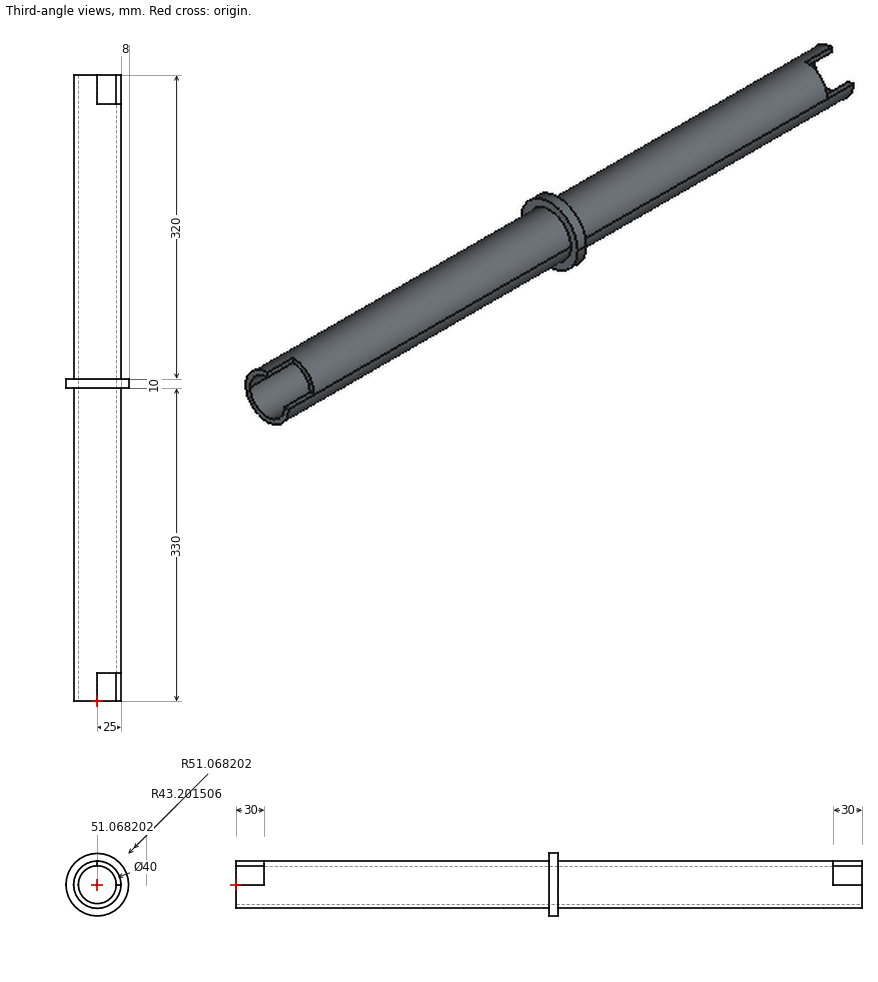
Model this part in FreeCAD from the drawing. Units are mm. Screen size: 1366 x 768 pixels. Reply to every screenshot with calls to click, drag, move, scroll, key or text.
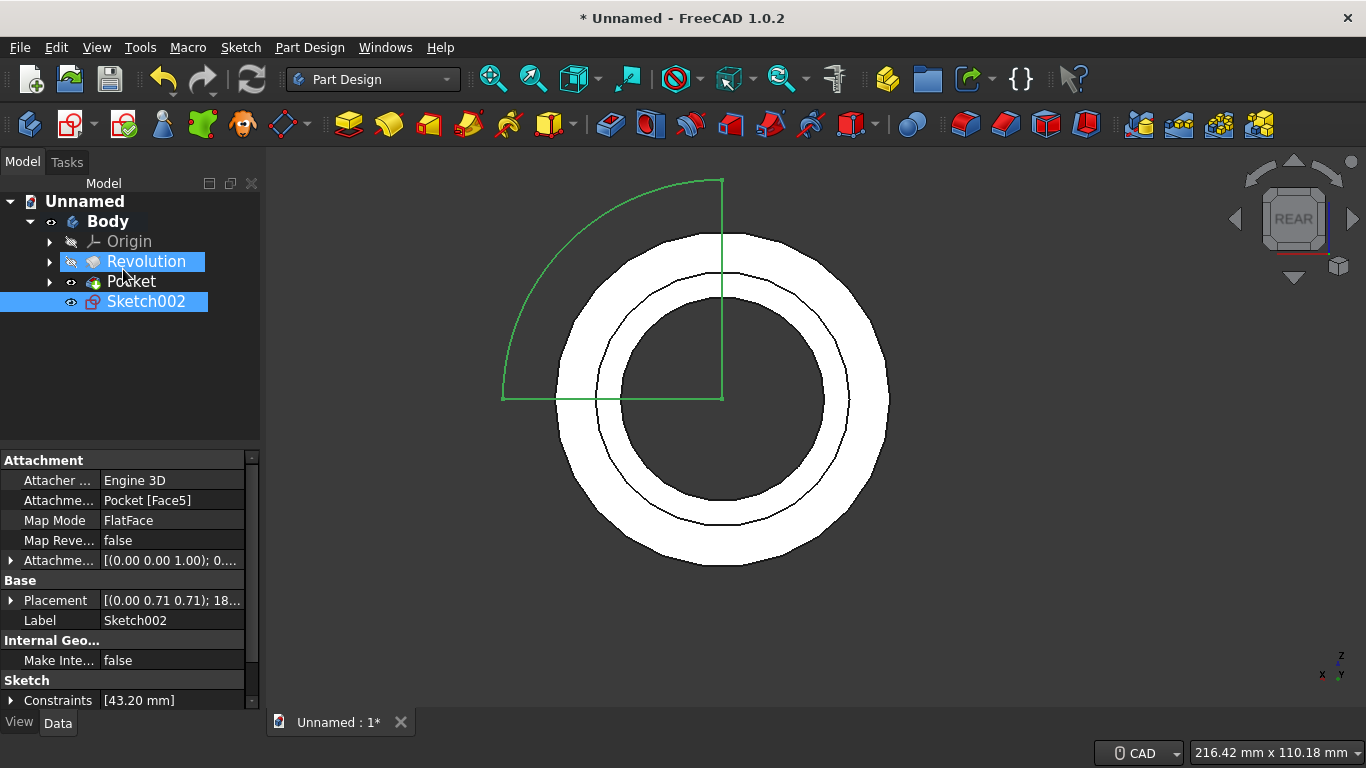
click(612, 124)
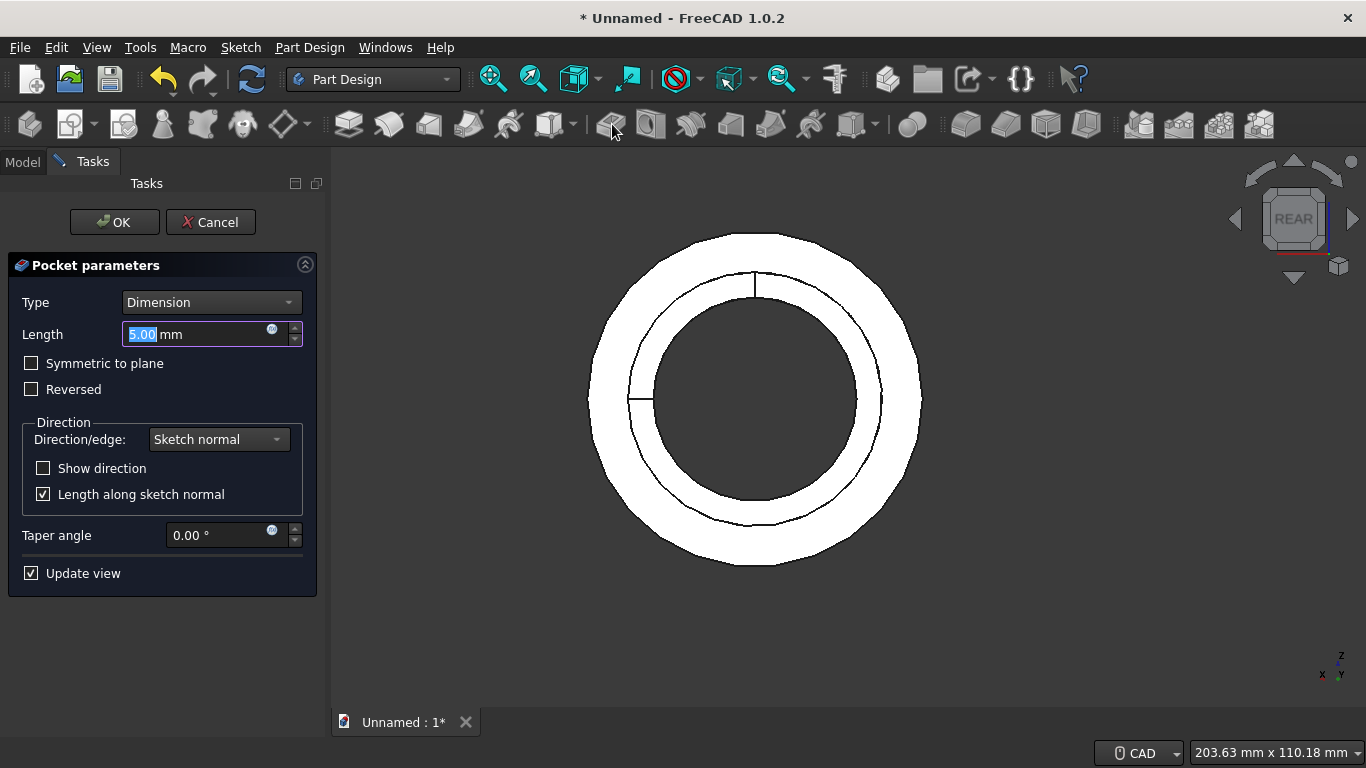
text(30)
key(Tab)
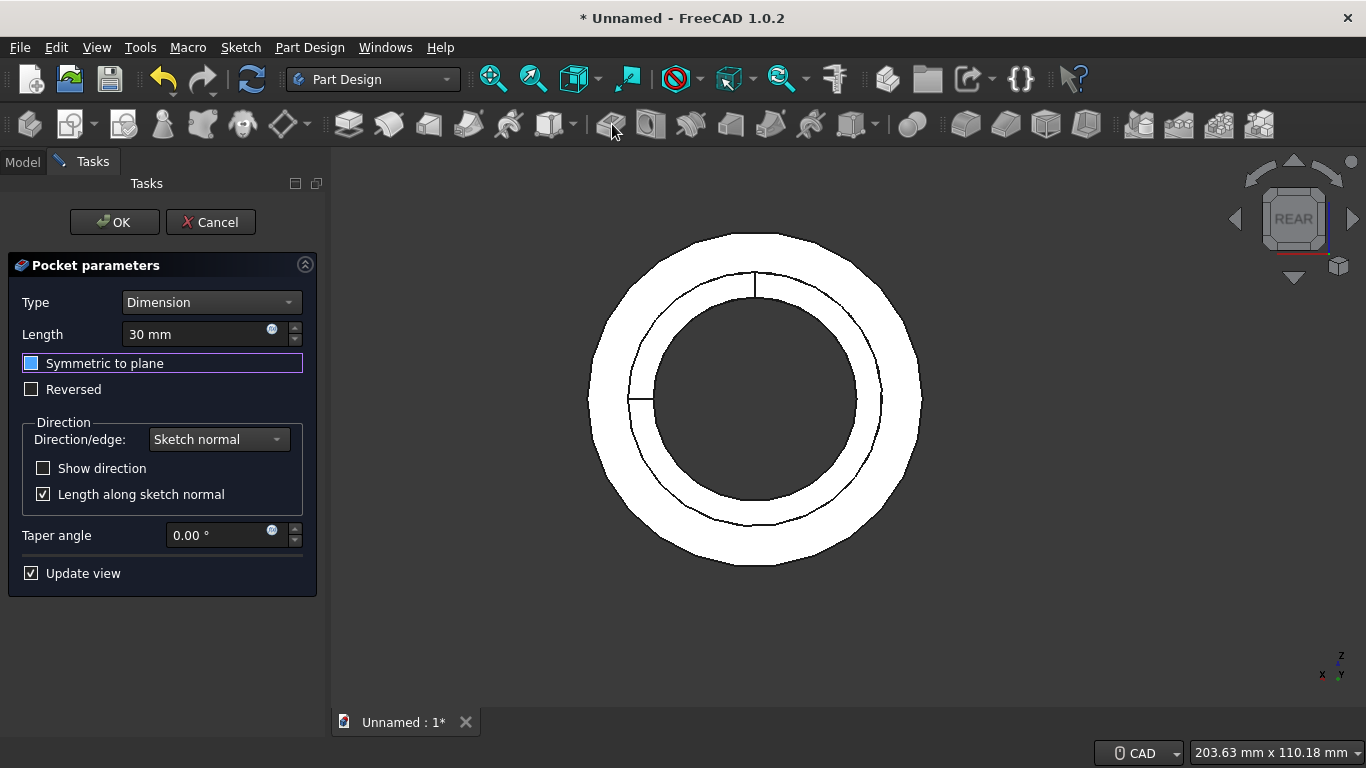
click(115, 222)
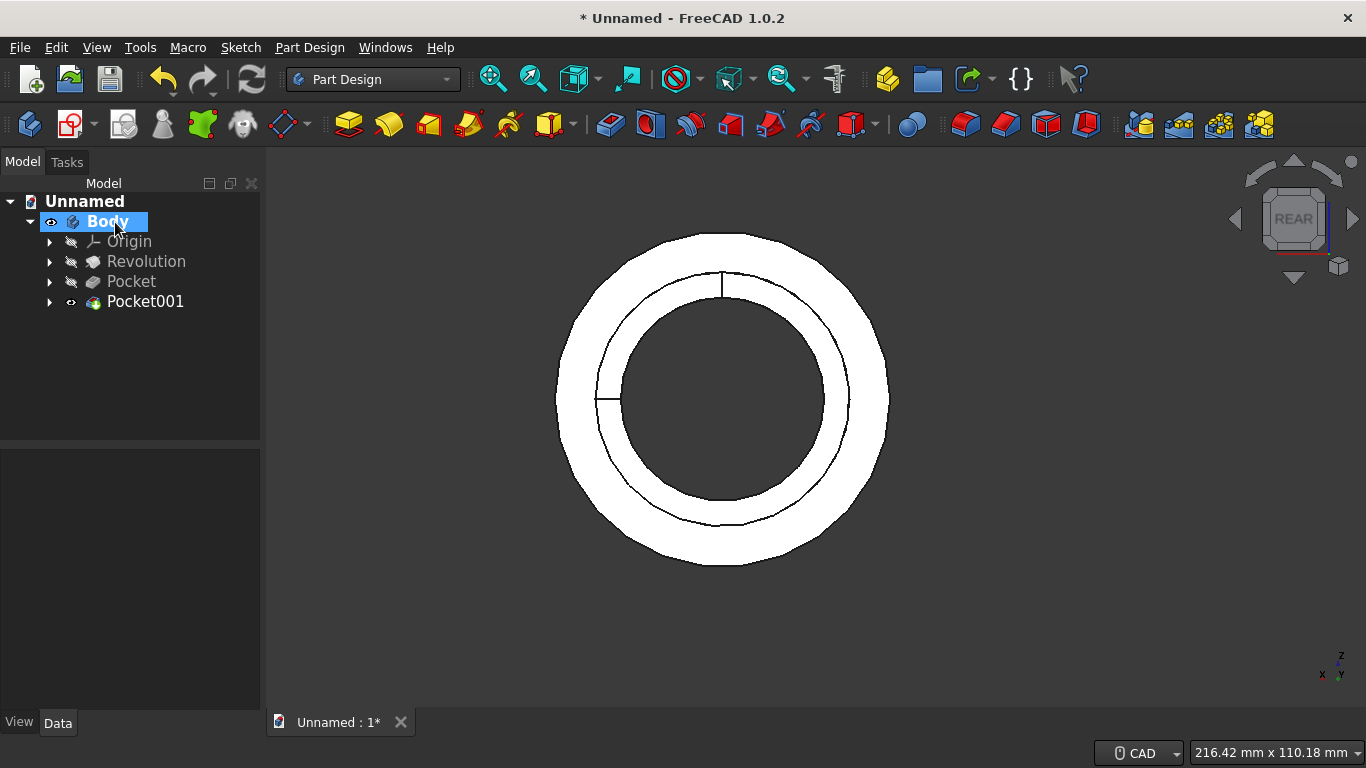
key(0)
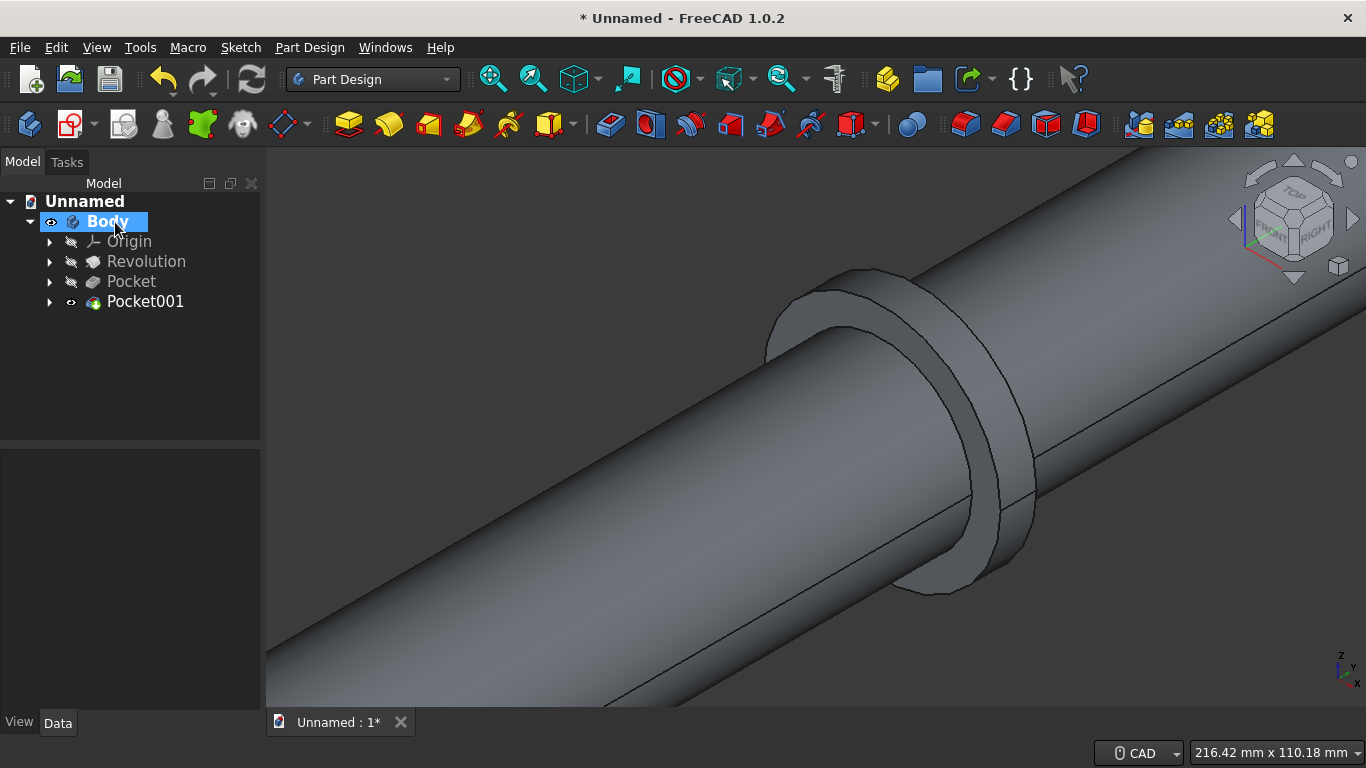
click(494, 80)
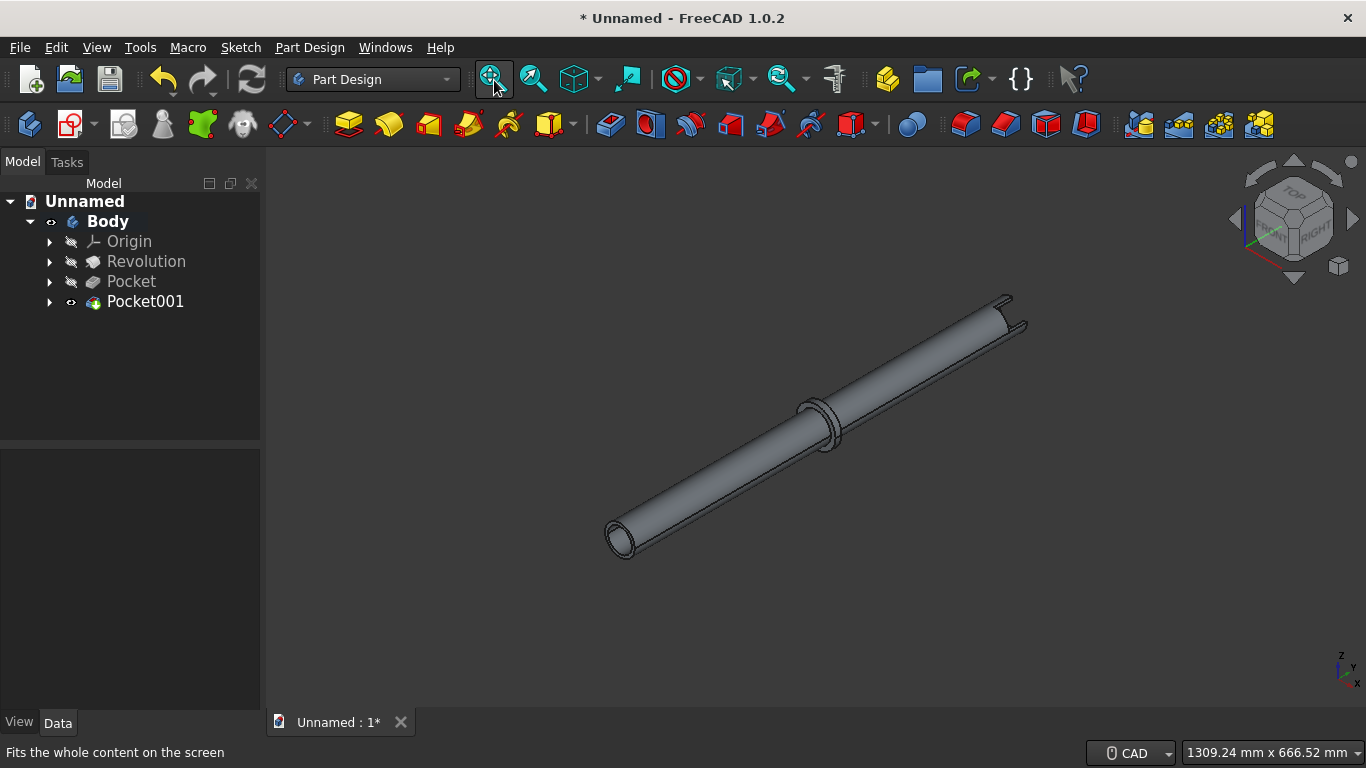
scroll(624, 556, up, 9)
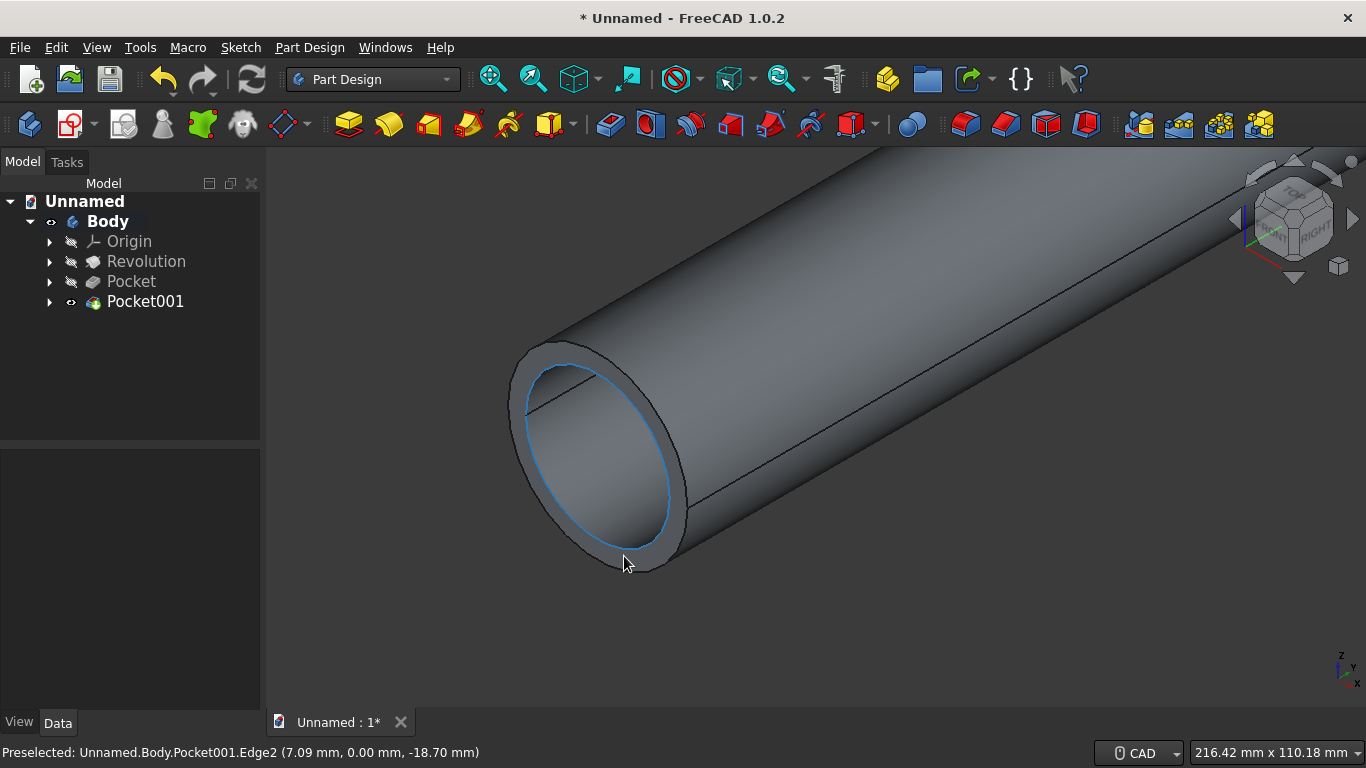
click(624, 559)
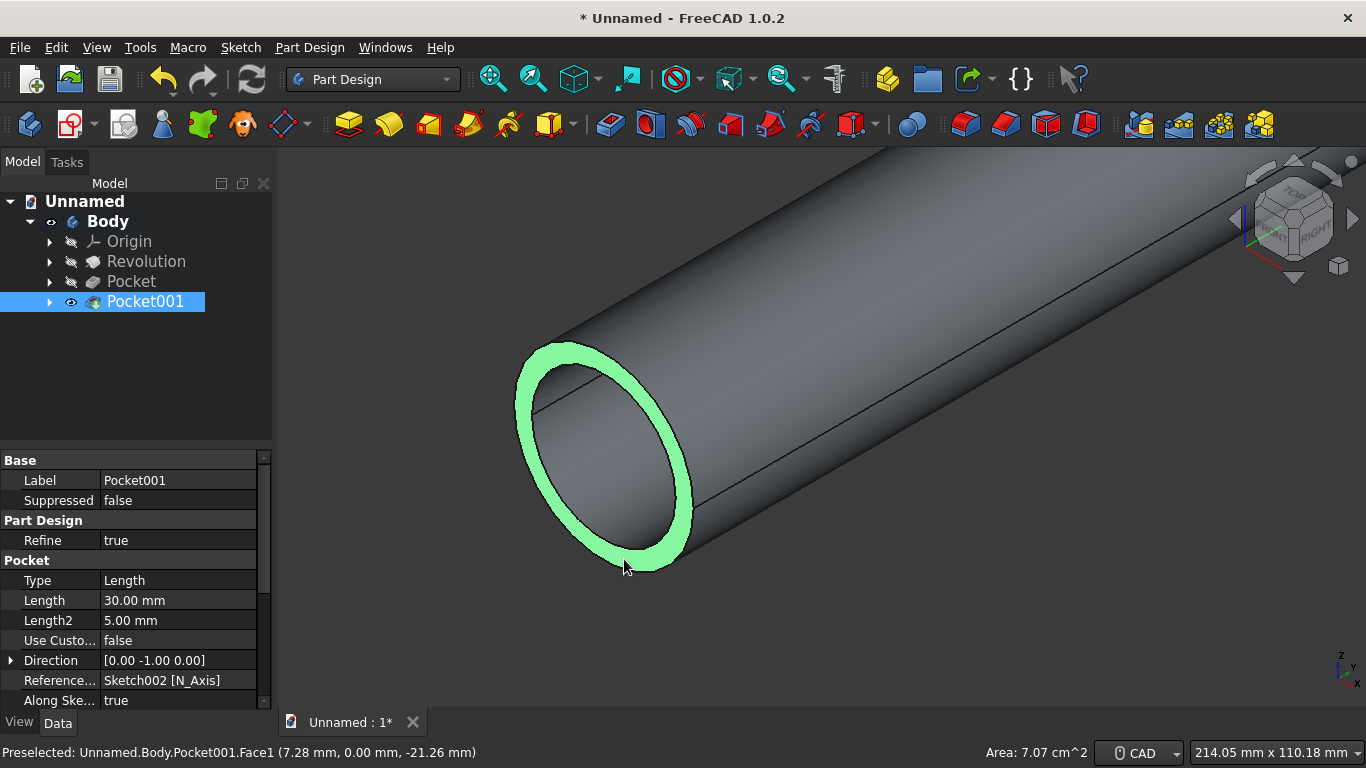
click(70, 124)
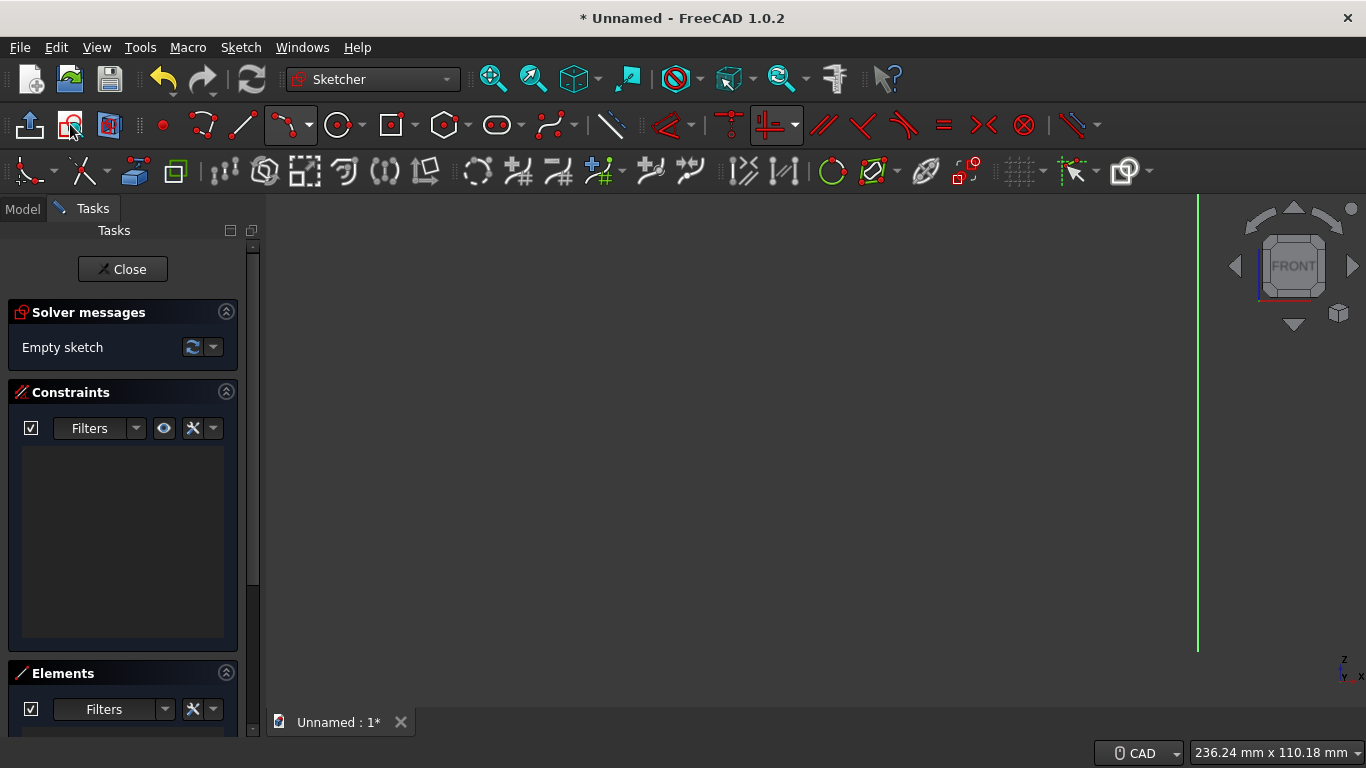
scroll(748, 450, down, 5)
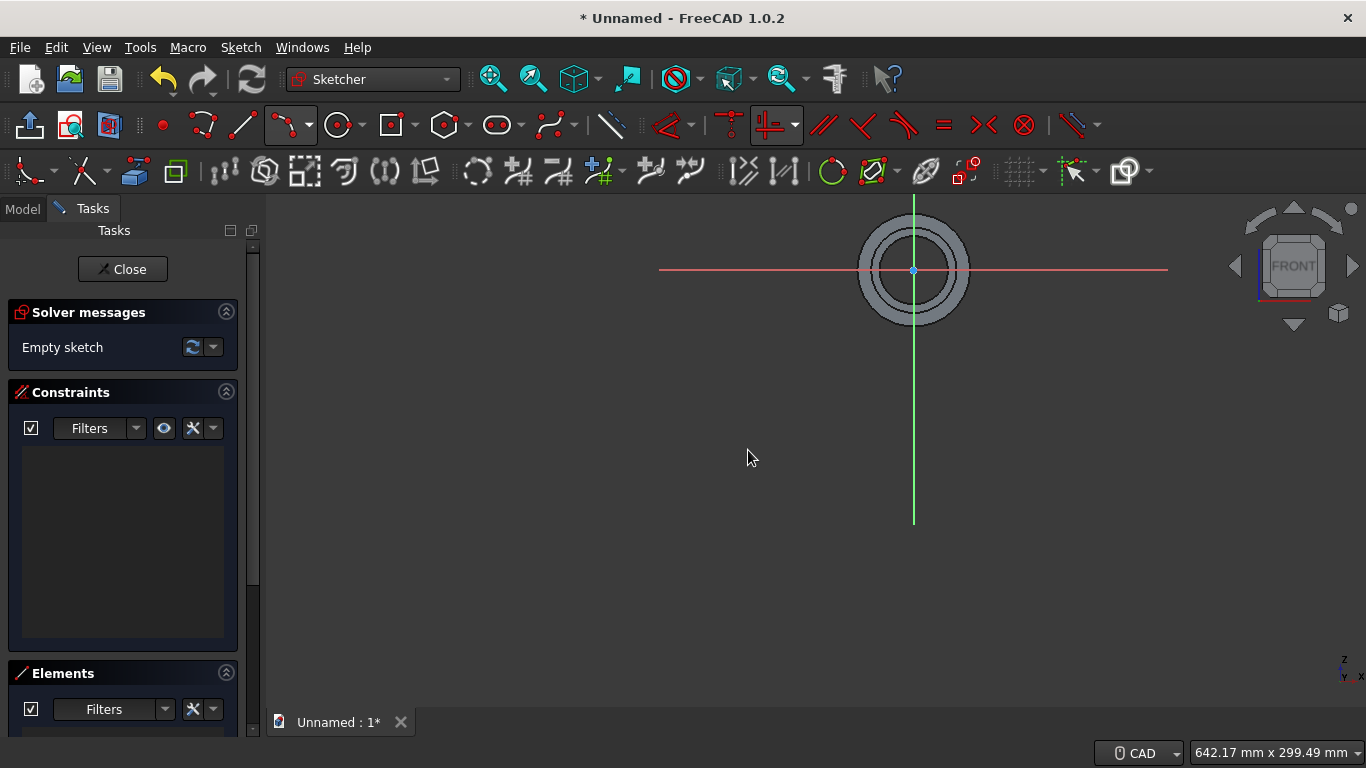
scroll(748, 450, down, 5)